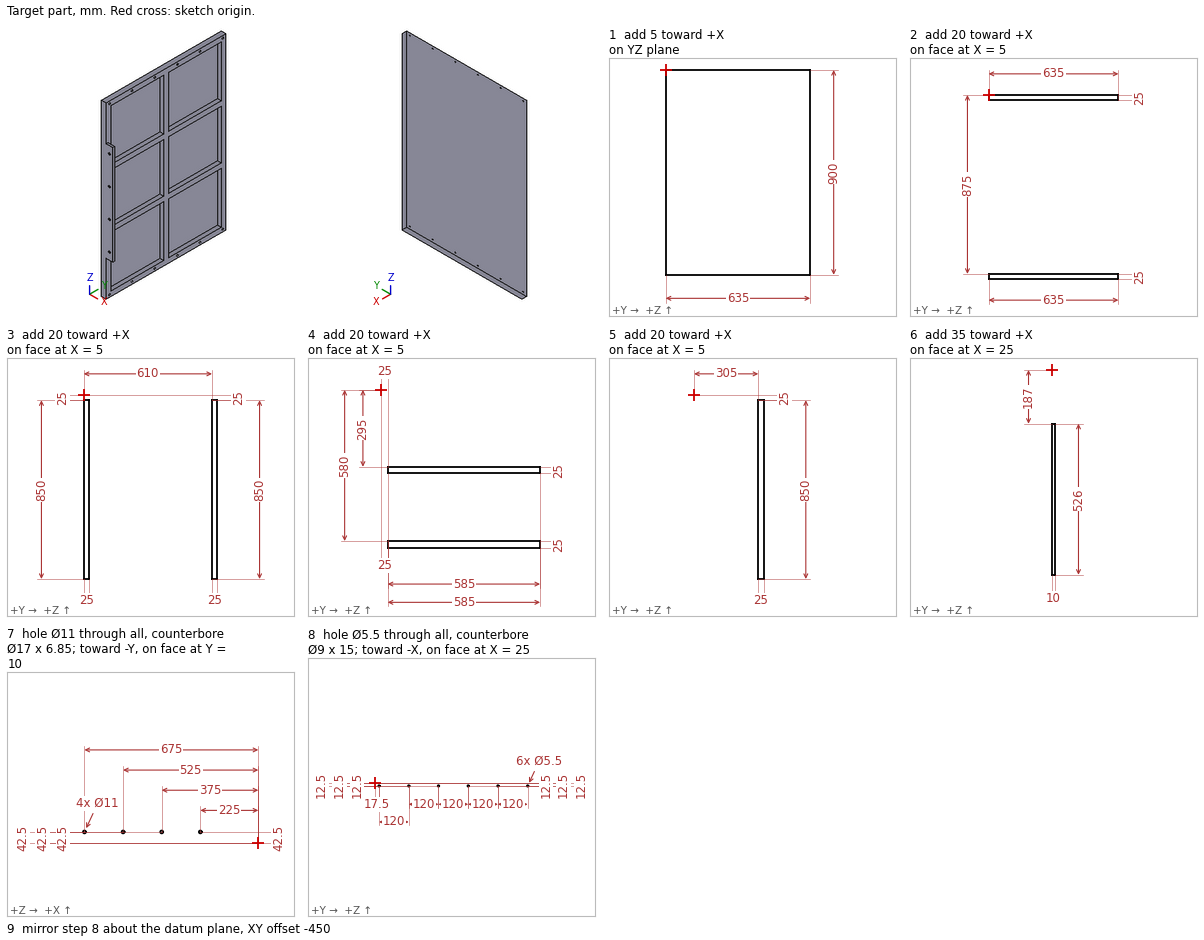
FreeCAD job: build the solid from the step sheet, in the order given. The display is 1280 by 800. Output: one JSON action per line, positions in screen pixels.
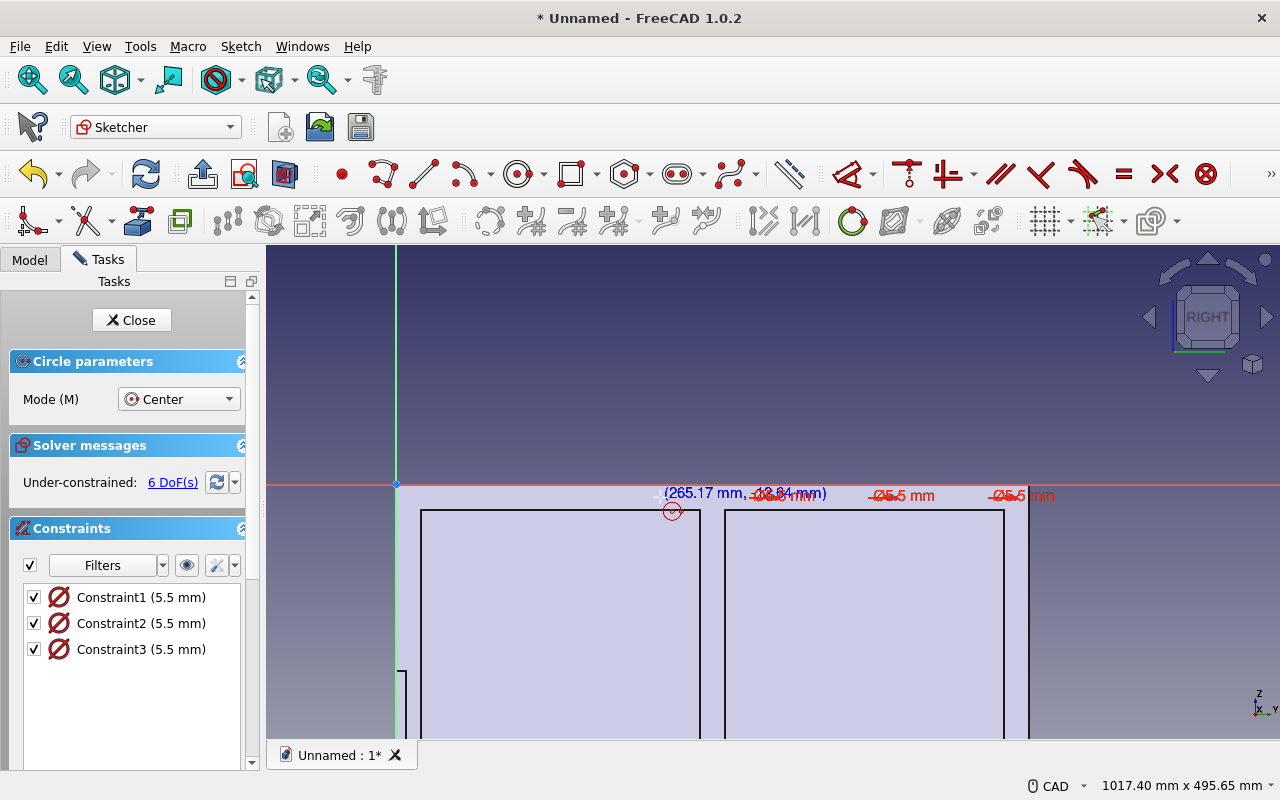
{"action": "scroll", "coordinate": [653, 497], "scroll_direction": "up", "scroll_amount": 2}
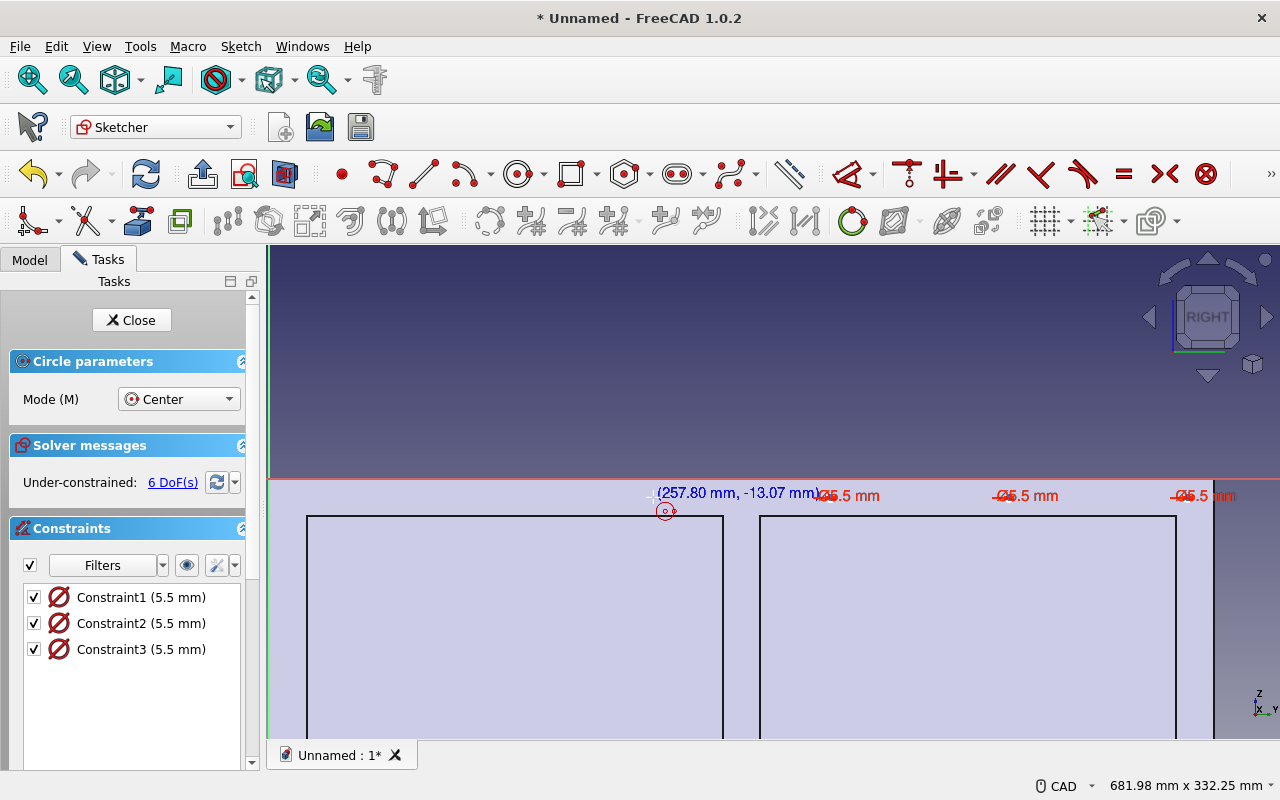
{"action": "left_click", "coordinate": [652, 497]}
{"action": "mouse_move", "coordinate": [655, 494]}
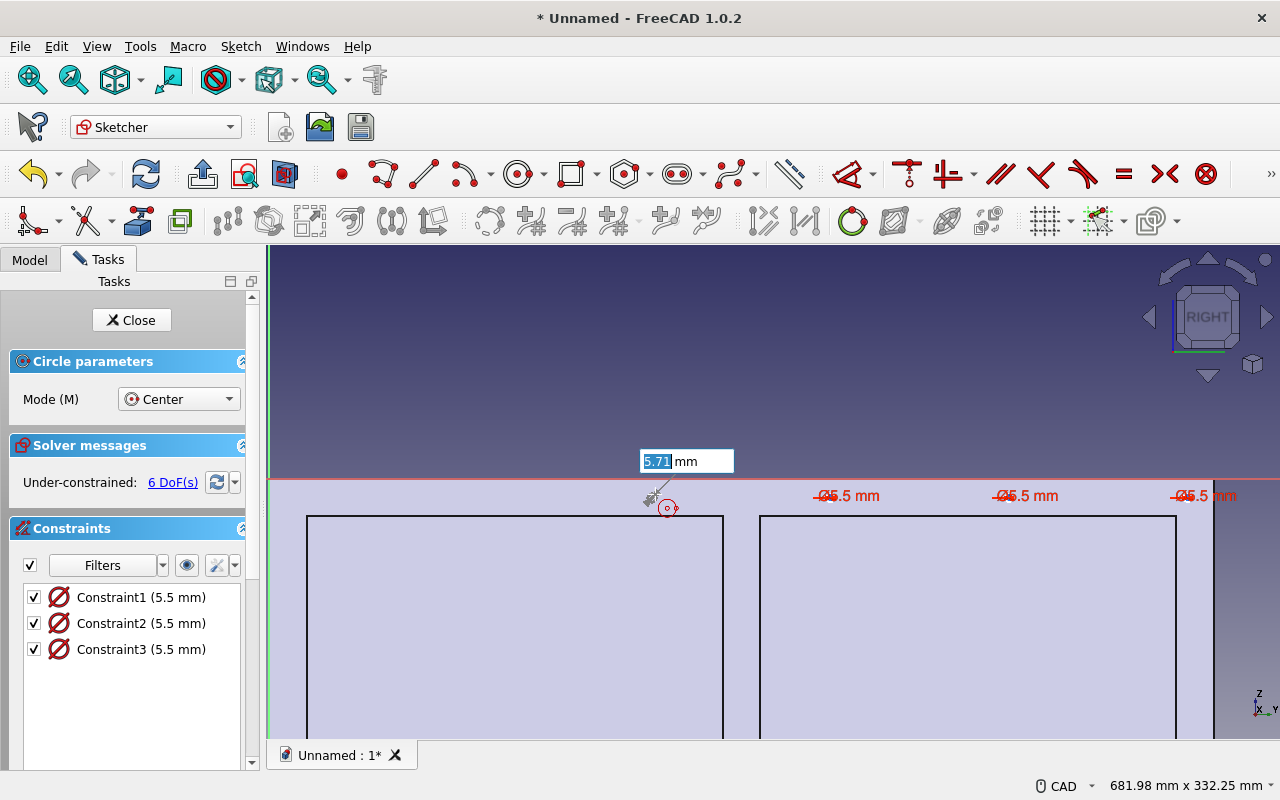
{"action": "type", "text": "5.5"}
{"action": "key", "text": "Return"}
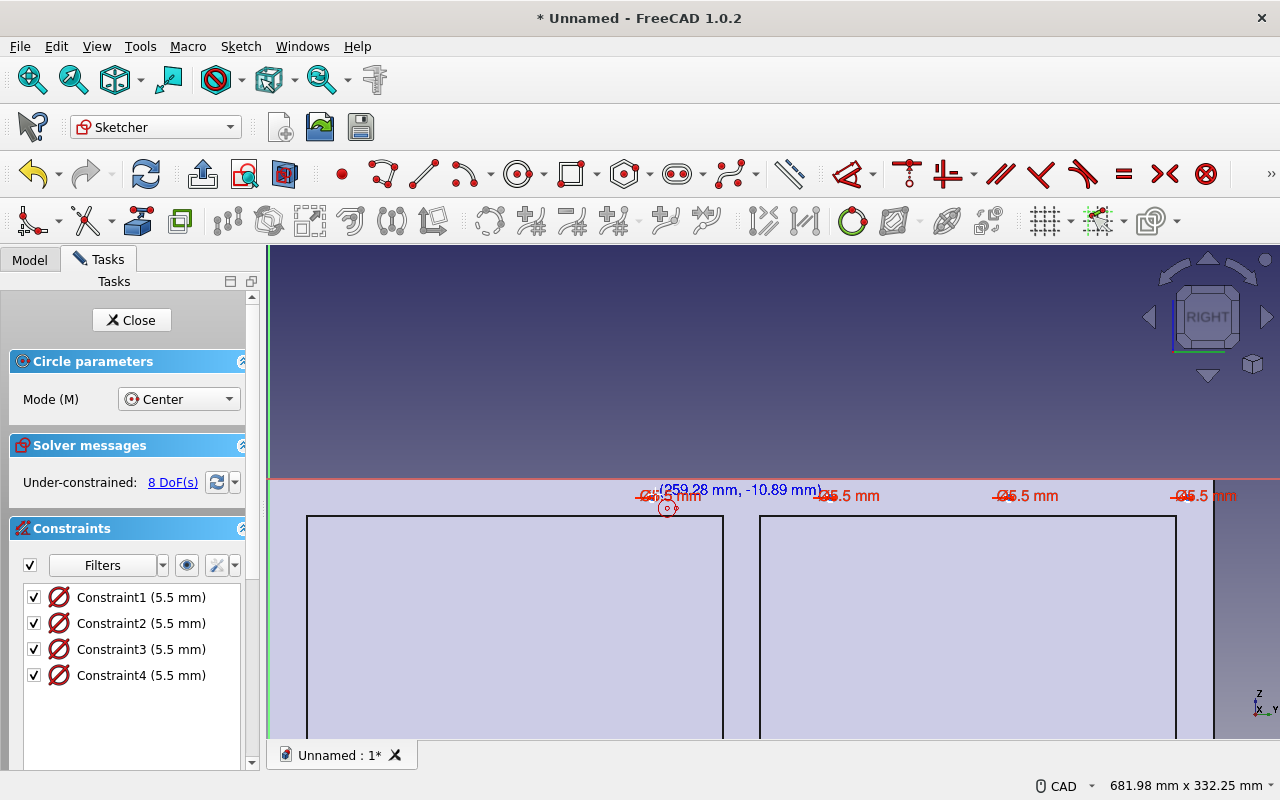
{"action": "scroll", "coordinate": [474, 497], "scroll_direction": "up", "scroll_amount": 9}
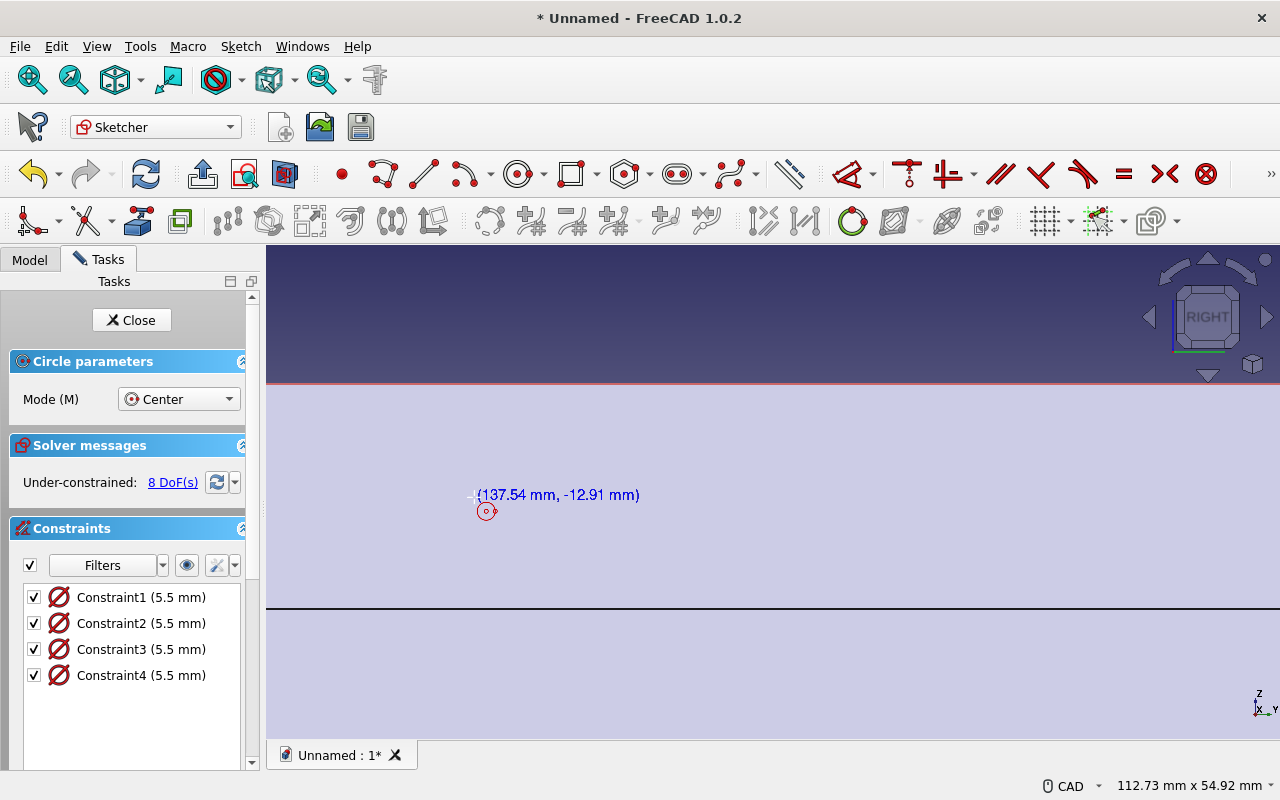
{"action": "scroll", "coordinate": [540, 497], "scroll_direction": "down", "scroll_amount": 11}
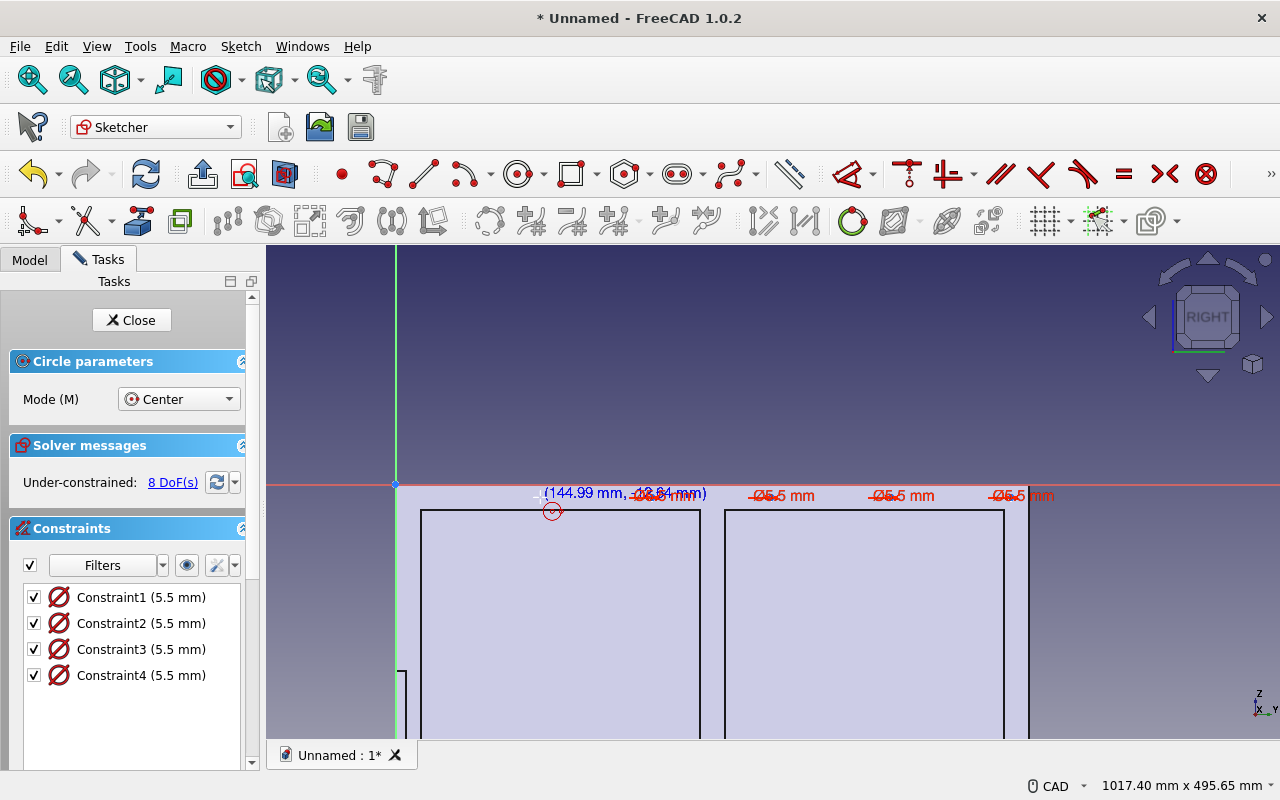
{"action": "scroll", "coordinate": [533, 497], "scroll_direction": "up", "scroll_amount": 2}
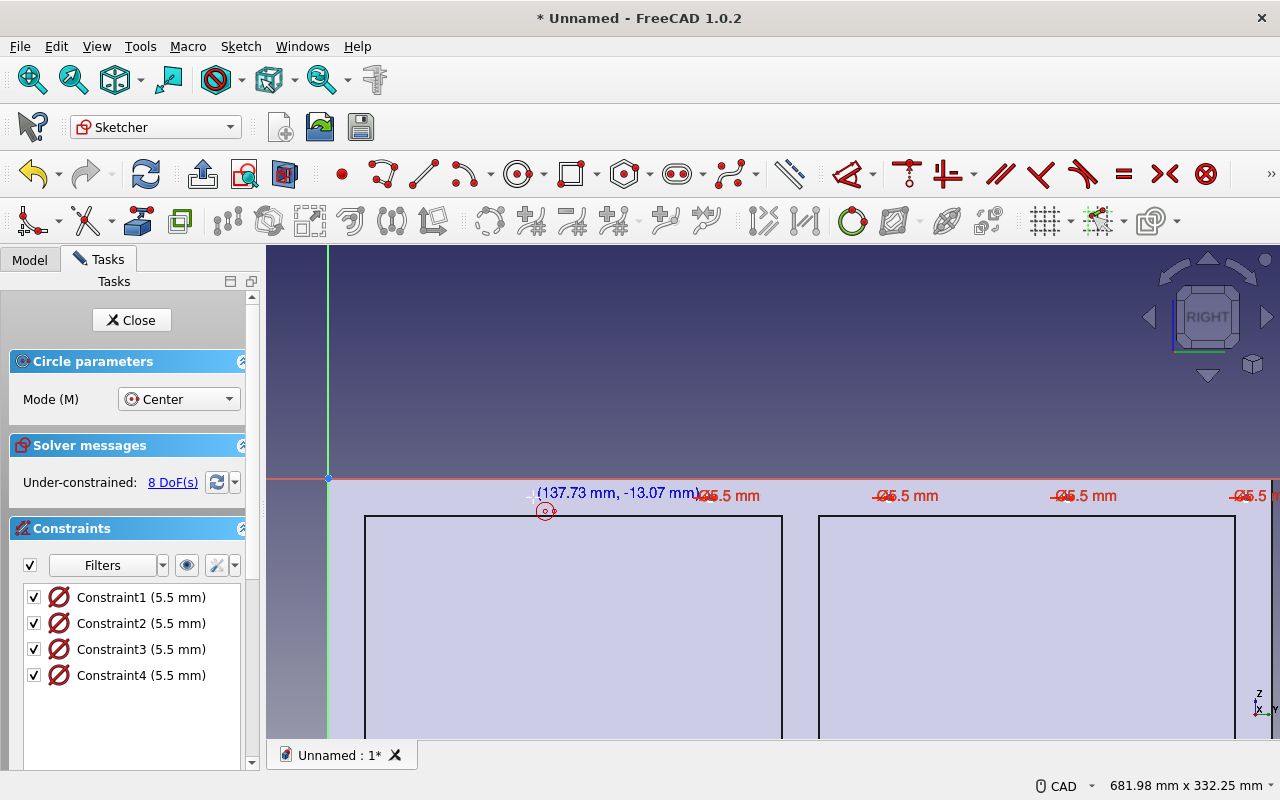
{"action": "left_click", "coordinate": [533, 497]}
{"action": "mouse_move", "coordinate": [535, 494]}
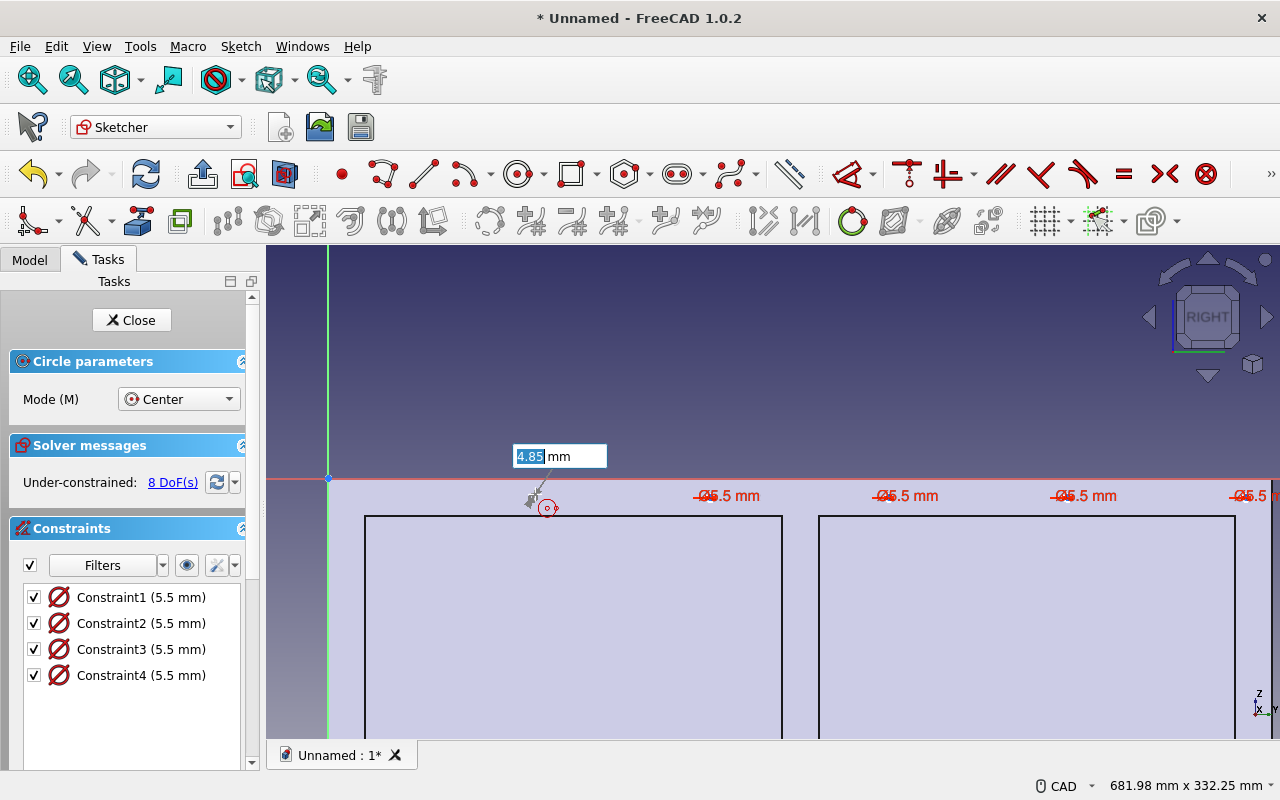
{"action": "type", "text": "5.5"}
{"action": "key", "text": "Return"}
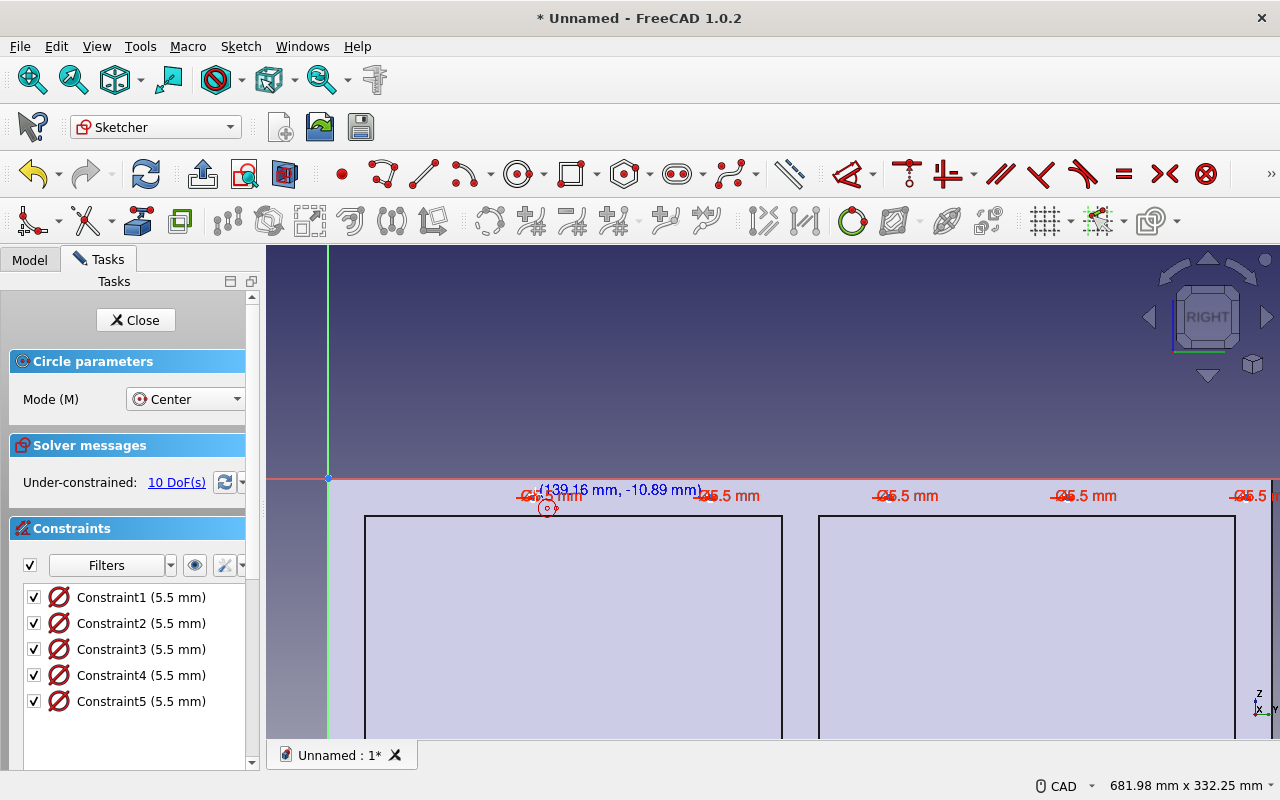
{"action": "scroll", "coordinate": [354, 497], "scroll_direction": "up", "scroll_amount": 9}